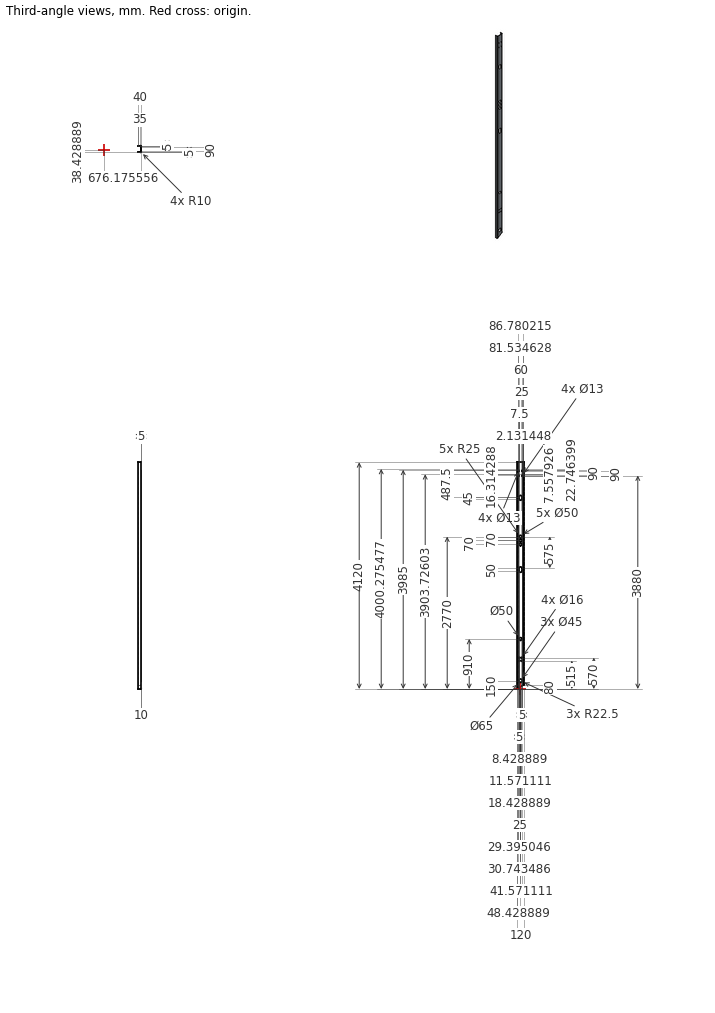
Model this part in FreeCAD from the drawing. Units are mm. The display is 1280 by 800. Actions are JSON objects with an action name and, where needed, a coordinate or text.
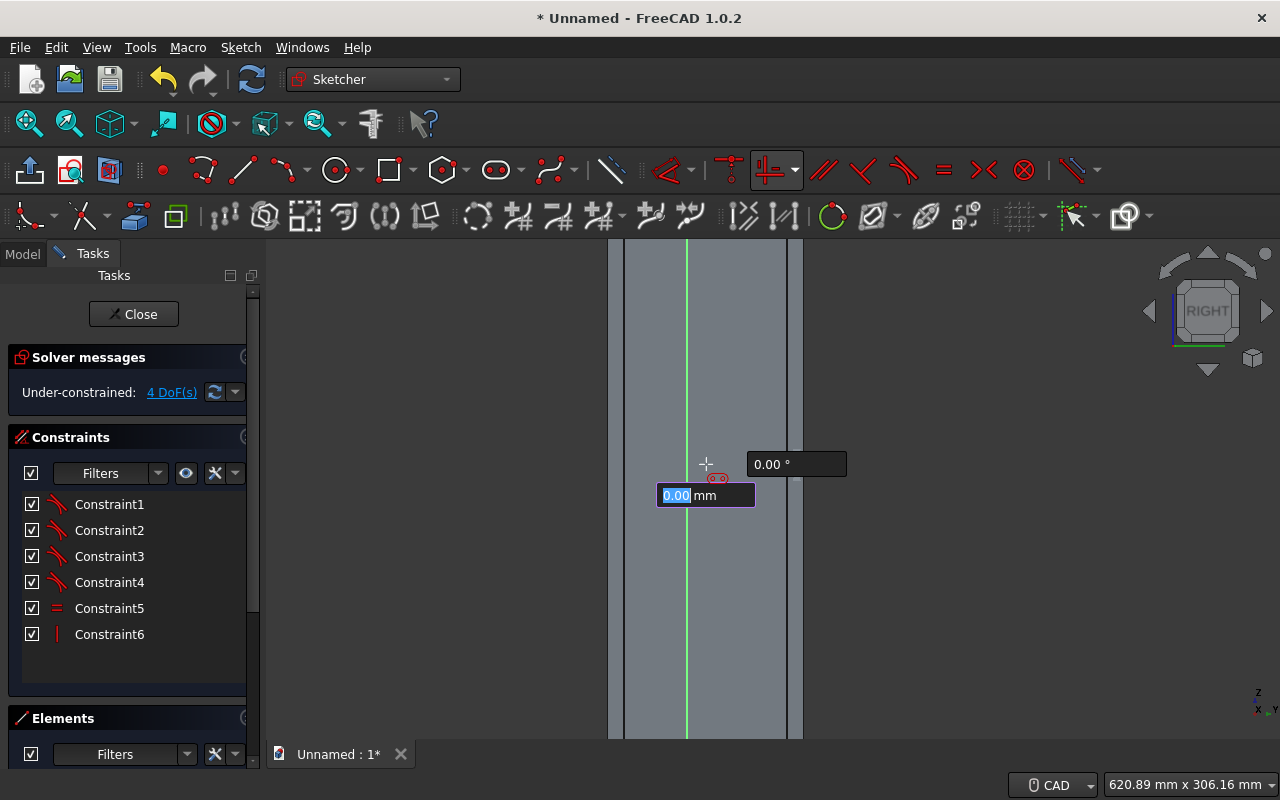
{"action": "left_click", "coordinate": [706, 382]}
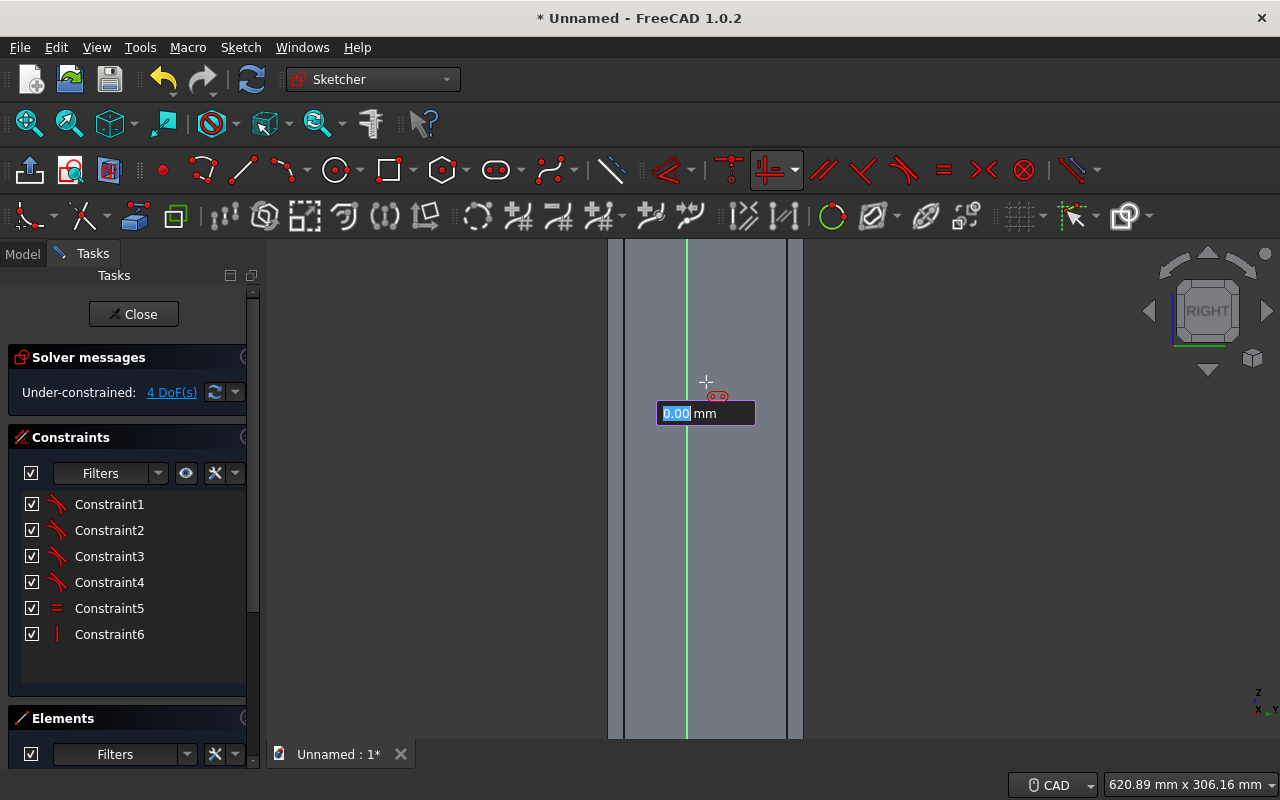
{"action": "left_click", "coordinate": [746, 423]}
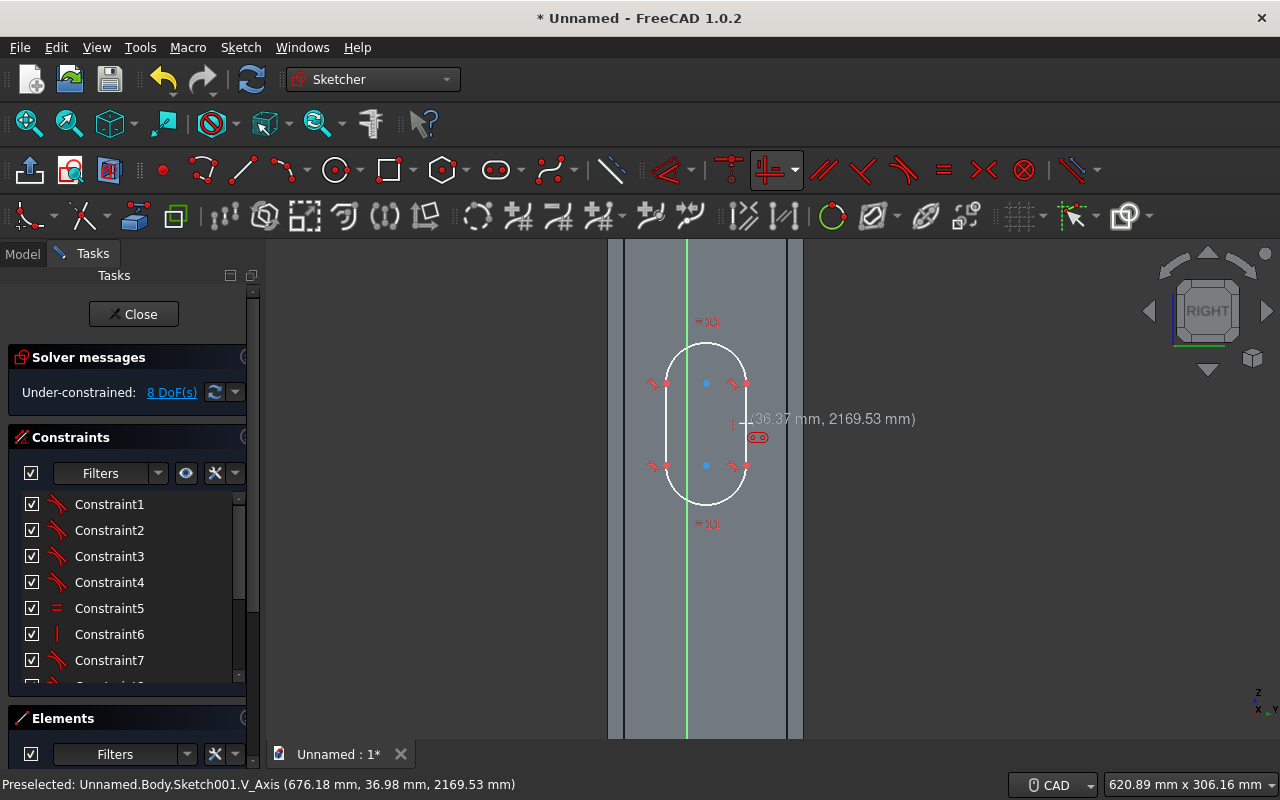
{"action": "key", "text": "g c"}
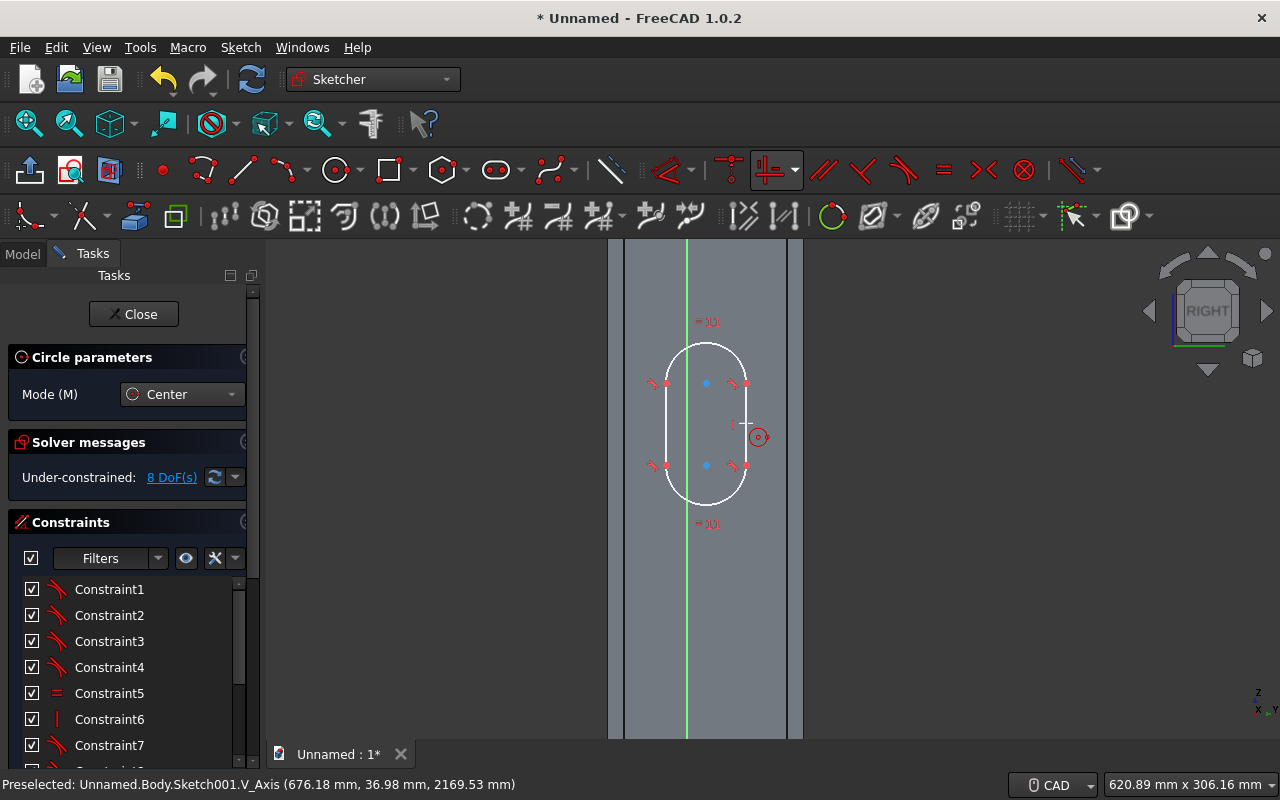
{"action": "scroll", "coordinate": [704, 478], "scroll_direction": "down", "scroll_amount": 15}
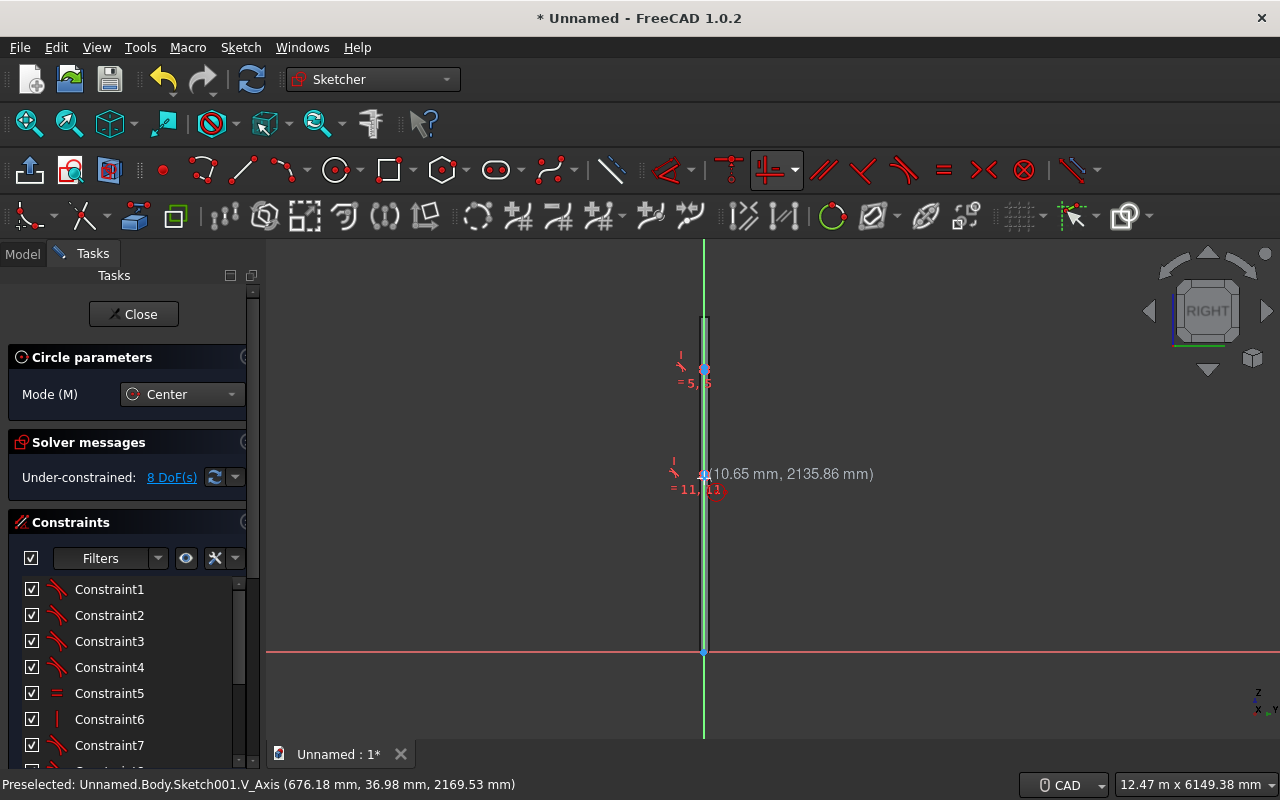
{"action": "scroll", "coordinate": [702, 328], "scroll_direction": "up", "scroll_amount": 19}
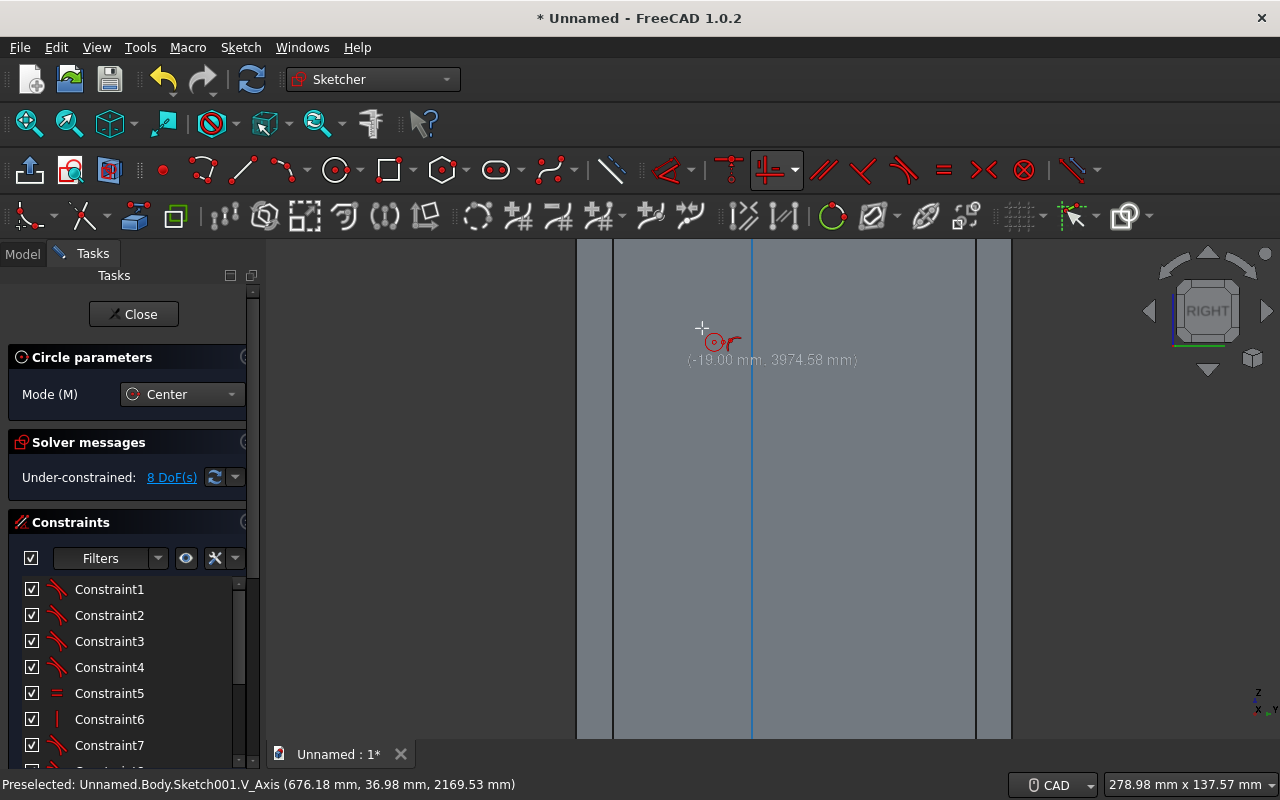
{"action": "scroll", "coordinate": [704, 489], "scroll_direction": "down", "scroll_amount": 15}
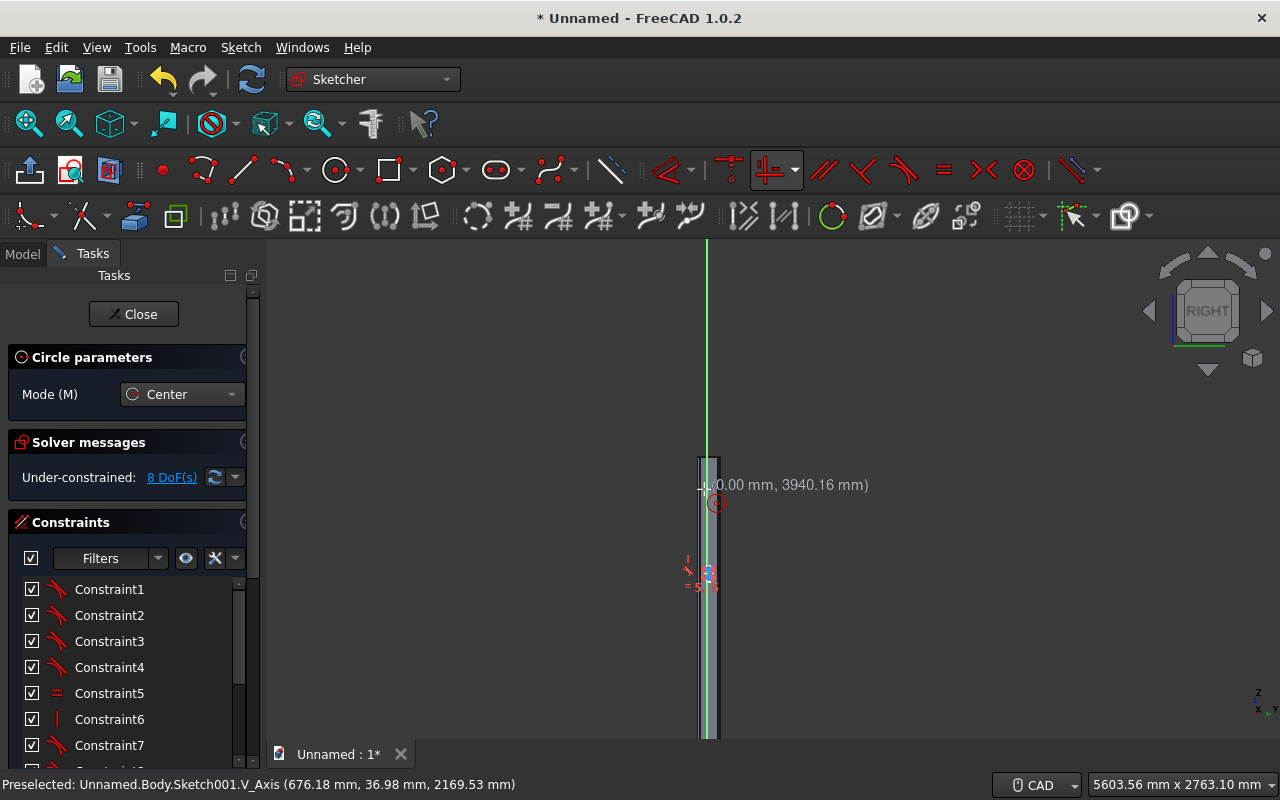
{"action": "scroll", "coordinate": [702, 284], "scroll_direction": "down", "scroll_amount": 5}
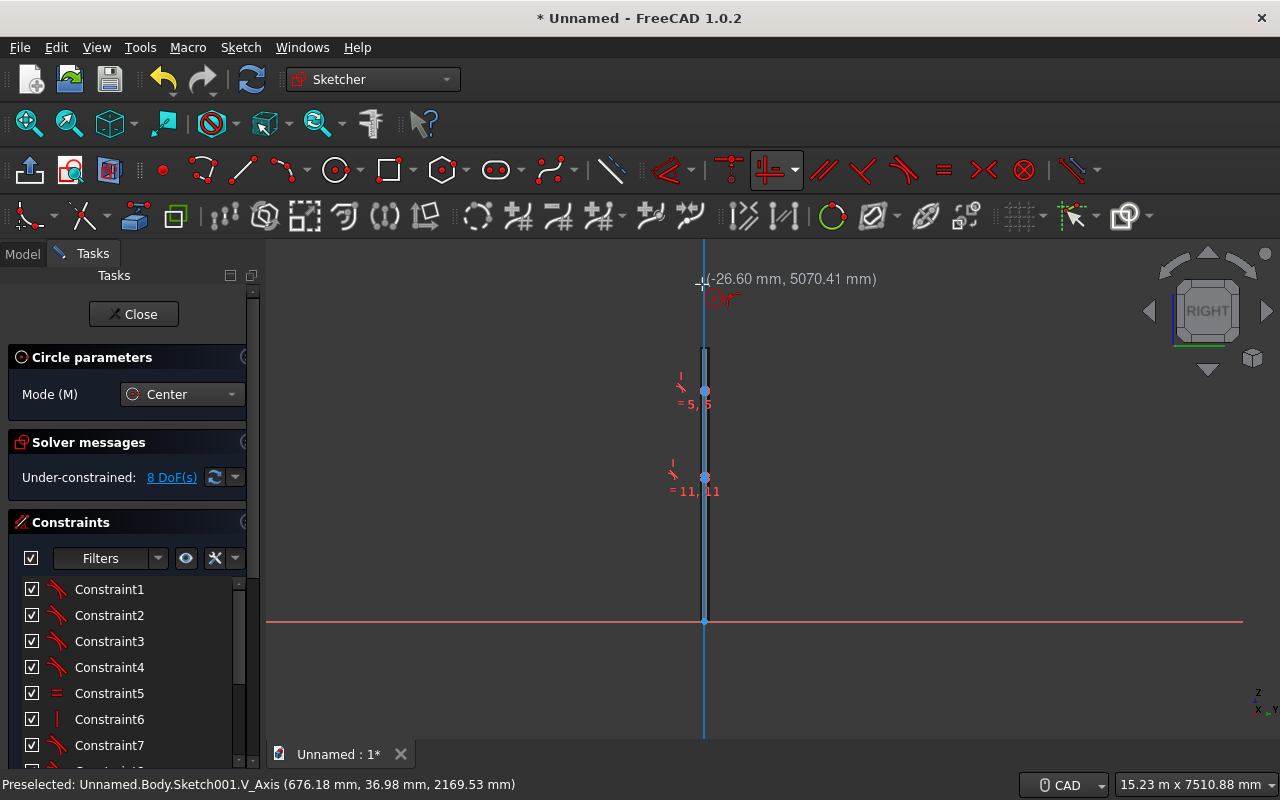
{"action": "scroll", "coordinate": [703, 357], "scroll_direction": "up", "scroll_amount": 13}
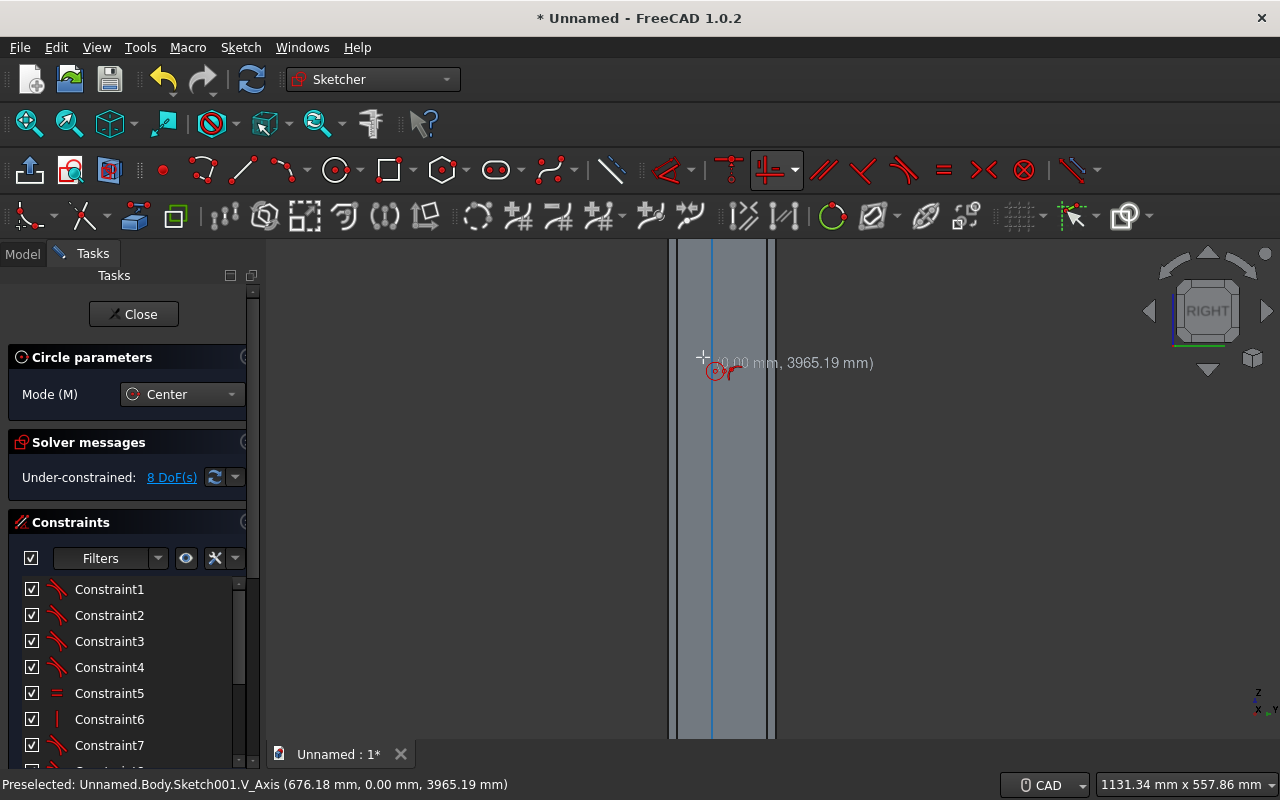
{"action": "left_click", "coordinate": [695, 350]}
{"action": "mouse_move", "coordinate": [691, 346]}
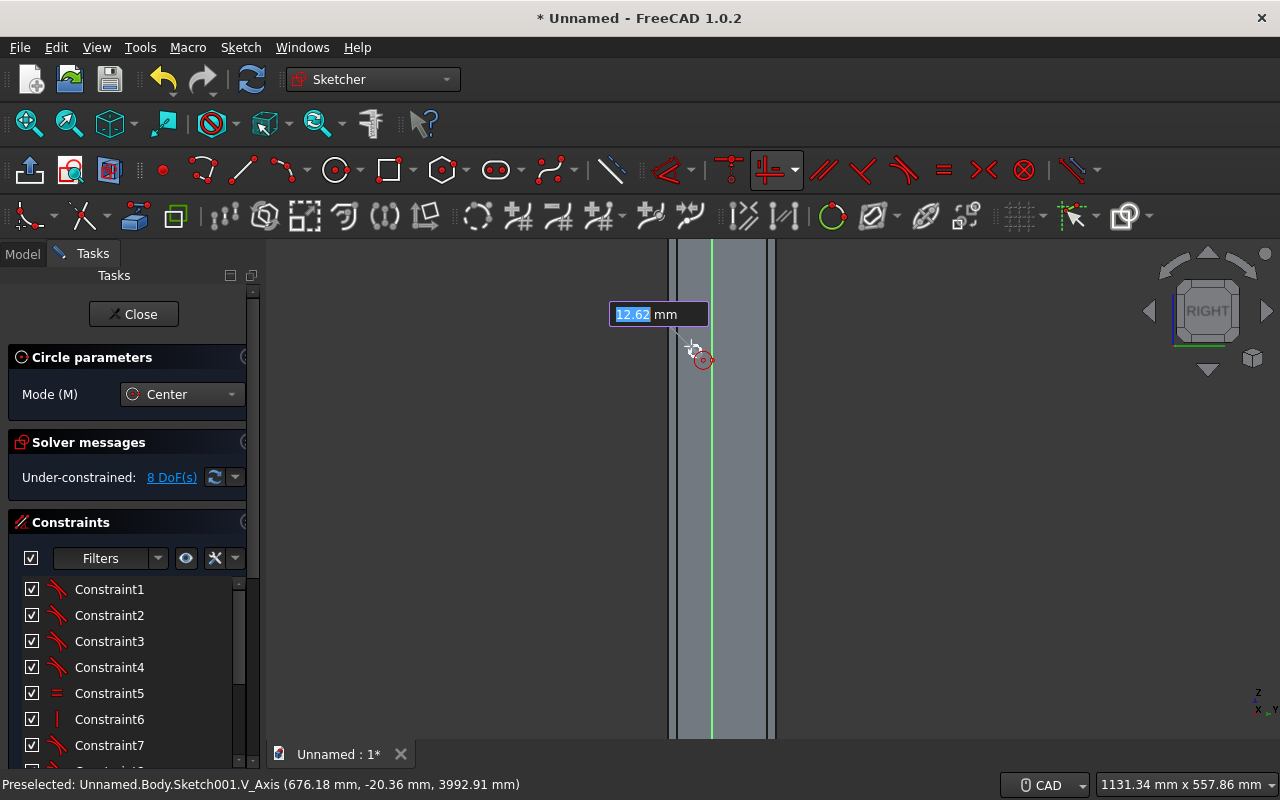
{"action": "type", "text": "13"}
{"action": "key", "text": "Return"}